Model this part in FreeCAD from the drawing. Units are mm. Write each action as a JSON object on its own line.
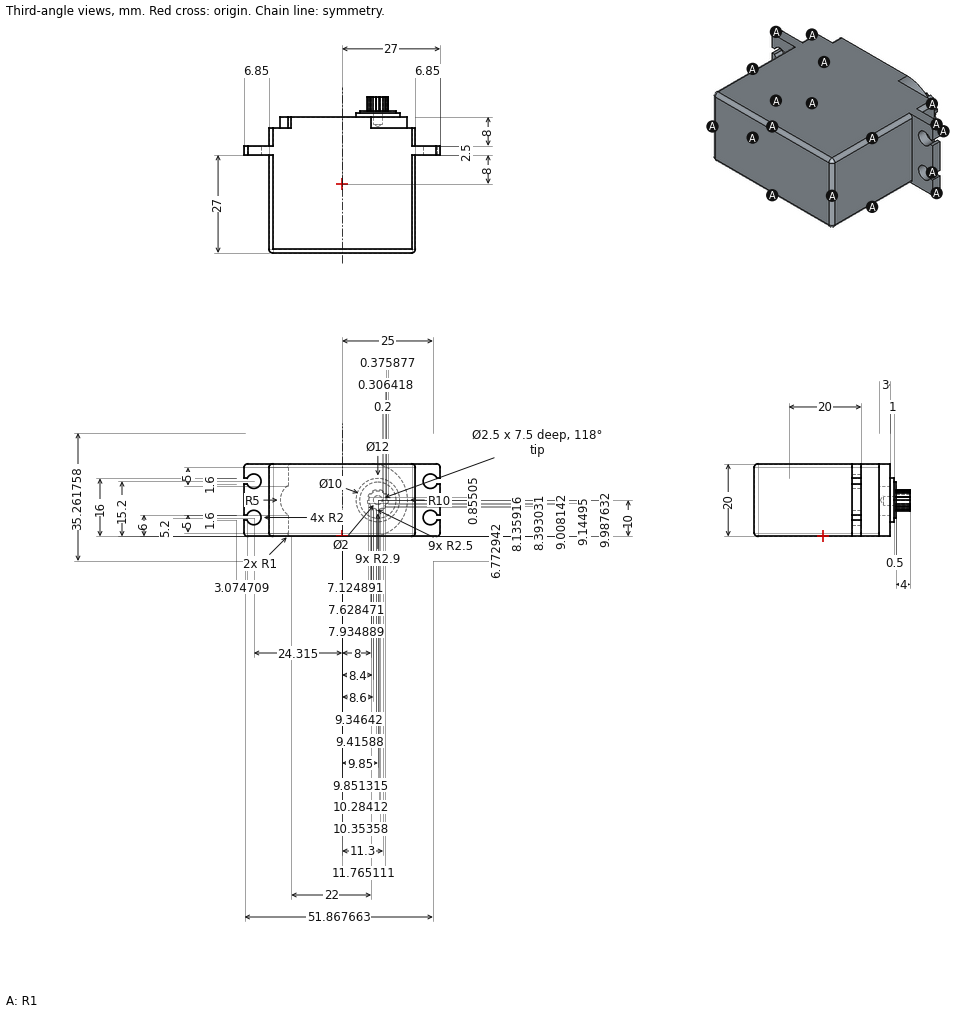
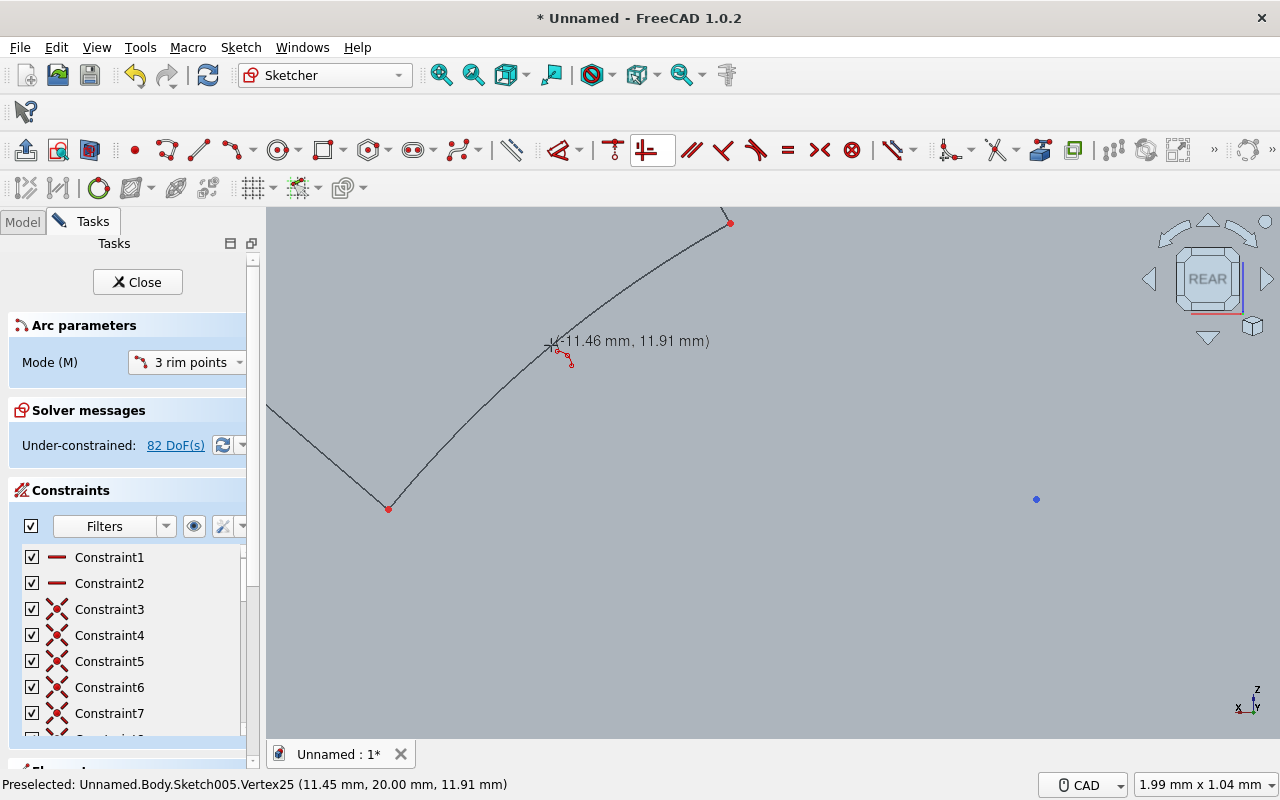
{"action": "scroll", "coordinate": [577, 333], "scroll_direction": "down", "scroll_amount": 15}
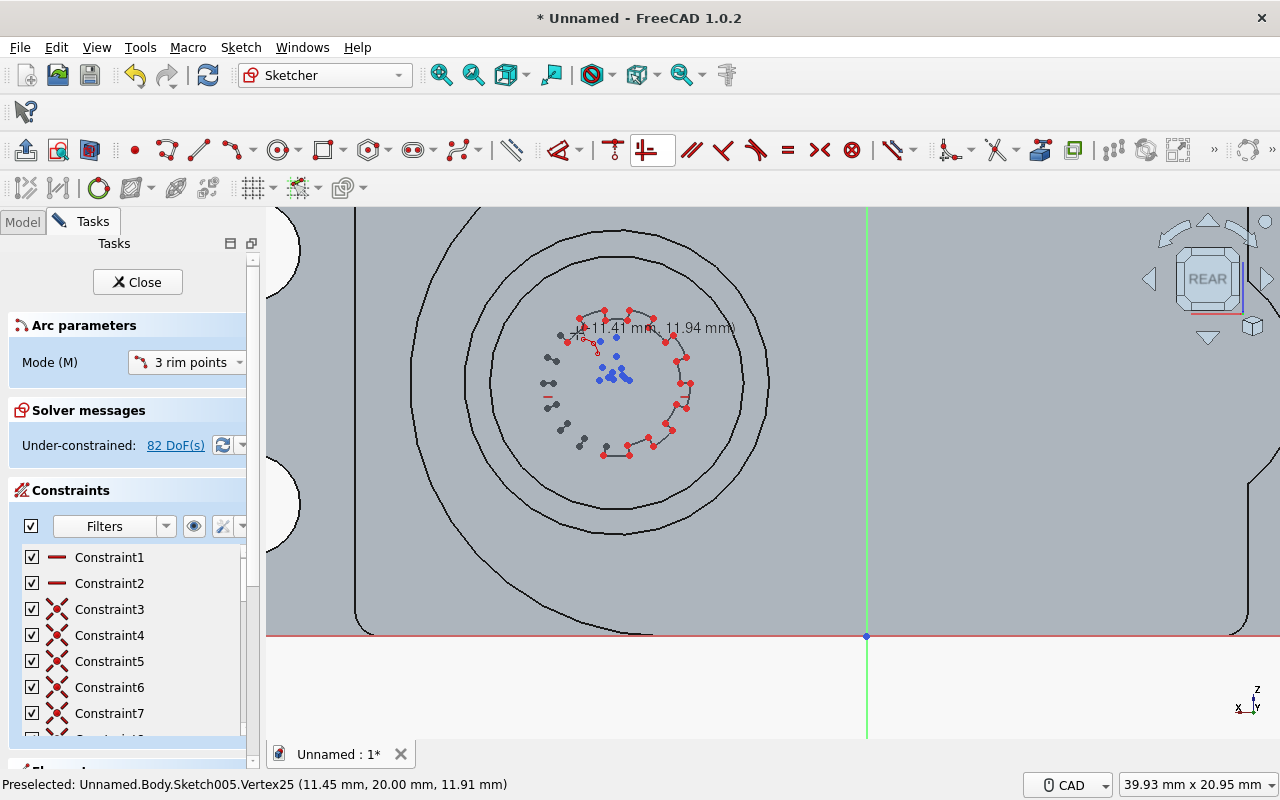
{"action": "scroll", "coordinate": [560, 335], "scroll_direction": "up", "scroll_amount": 6}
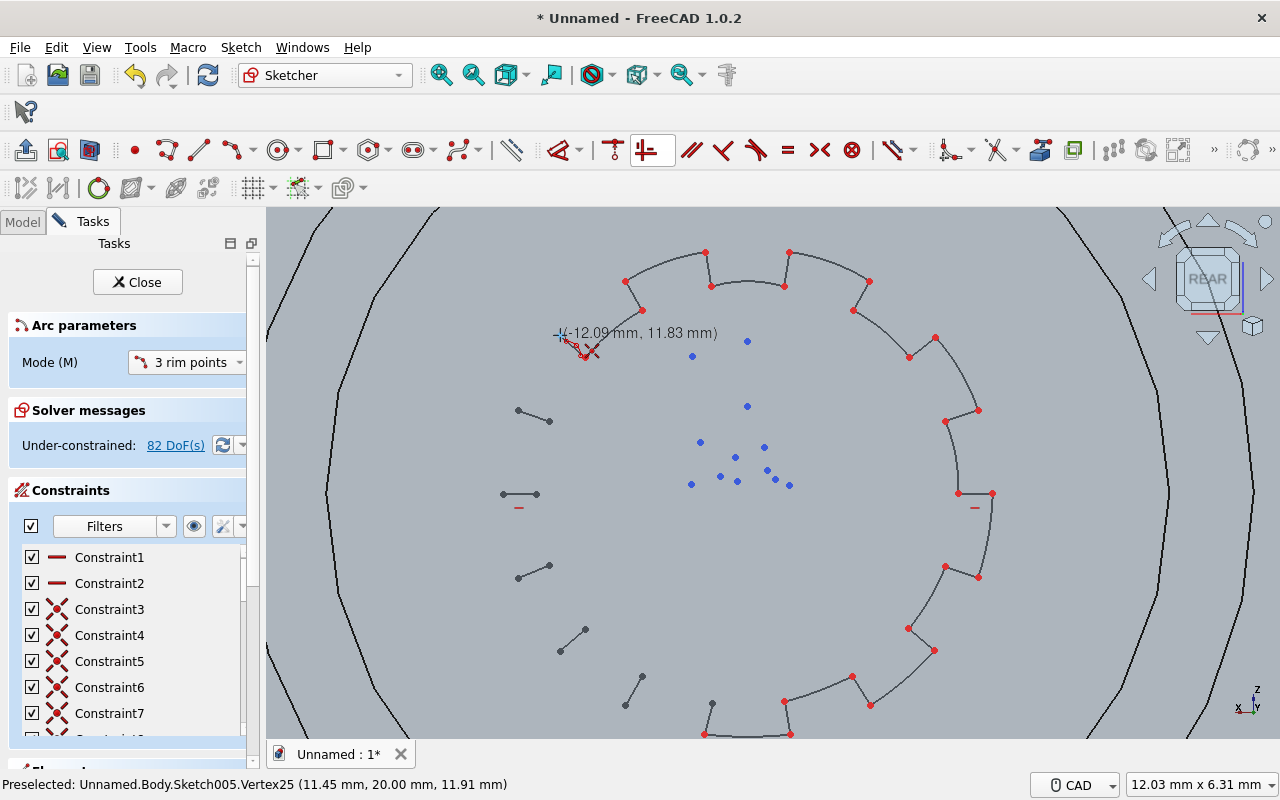
{"action": "left_click", "coordinate": [560, 336]}
{"action": "left_click", "coordinate": [518, 411]}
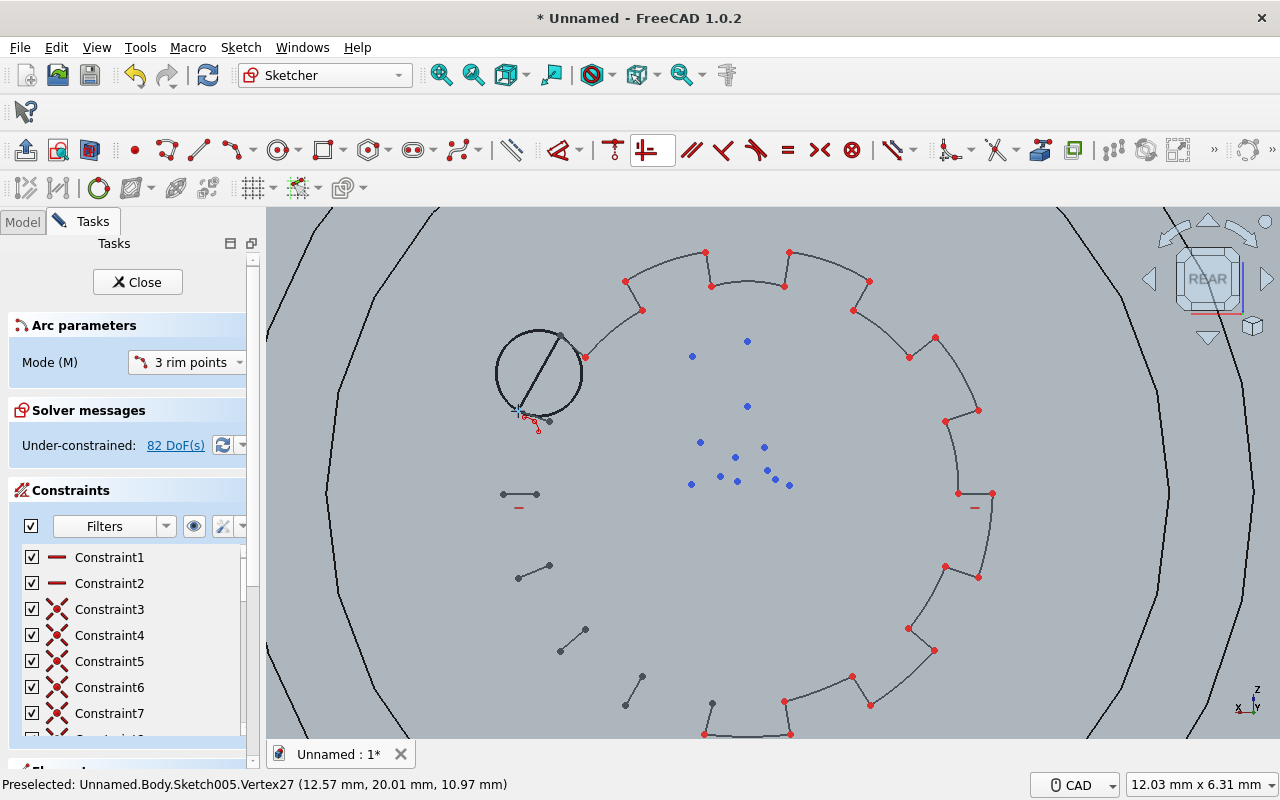
{"action": "scroll", "coordinate": [536, 370], "scroll_direction": "up", "scroll_amount": 8}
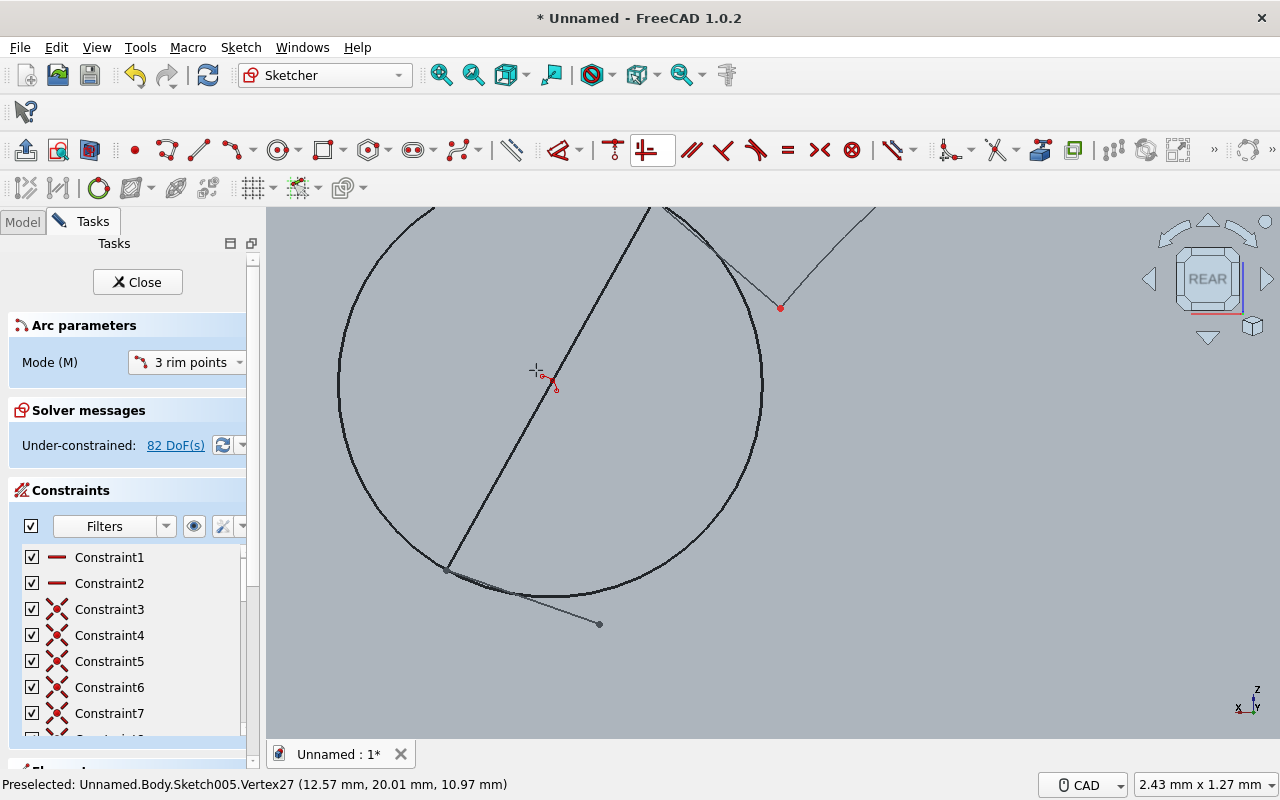
{"action": "left_click", "coordinate": [536, 368]}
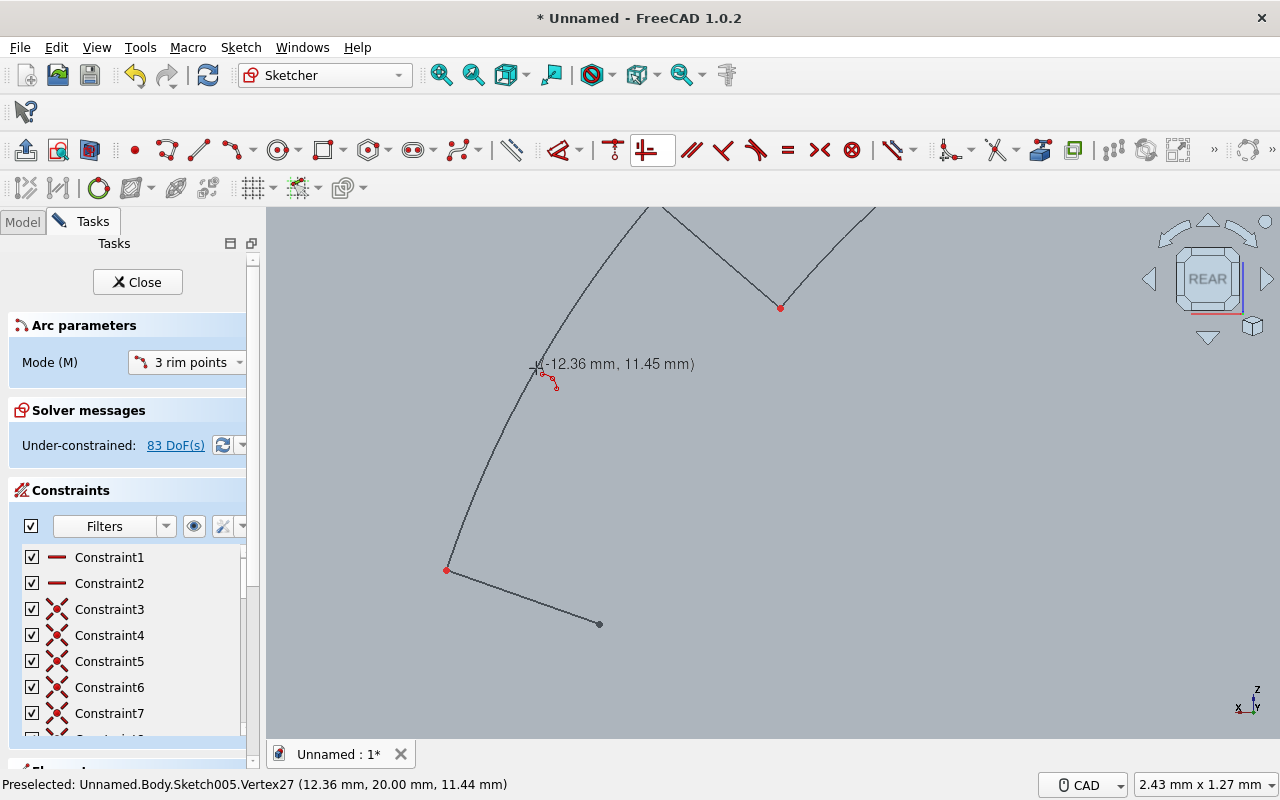
{"action": "scroll", "coordinate": [554, 344], "scroll_direction": "down", "scroll_amount": 14}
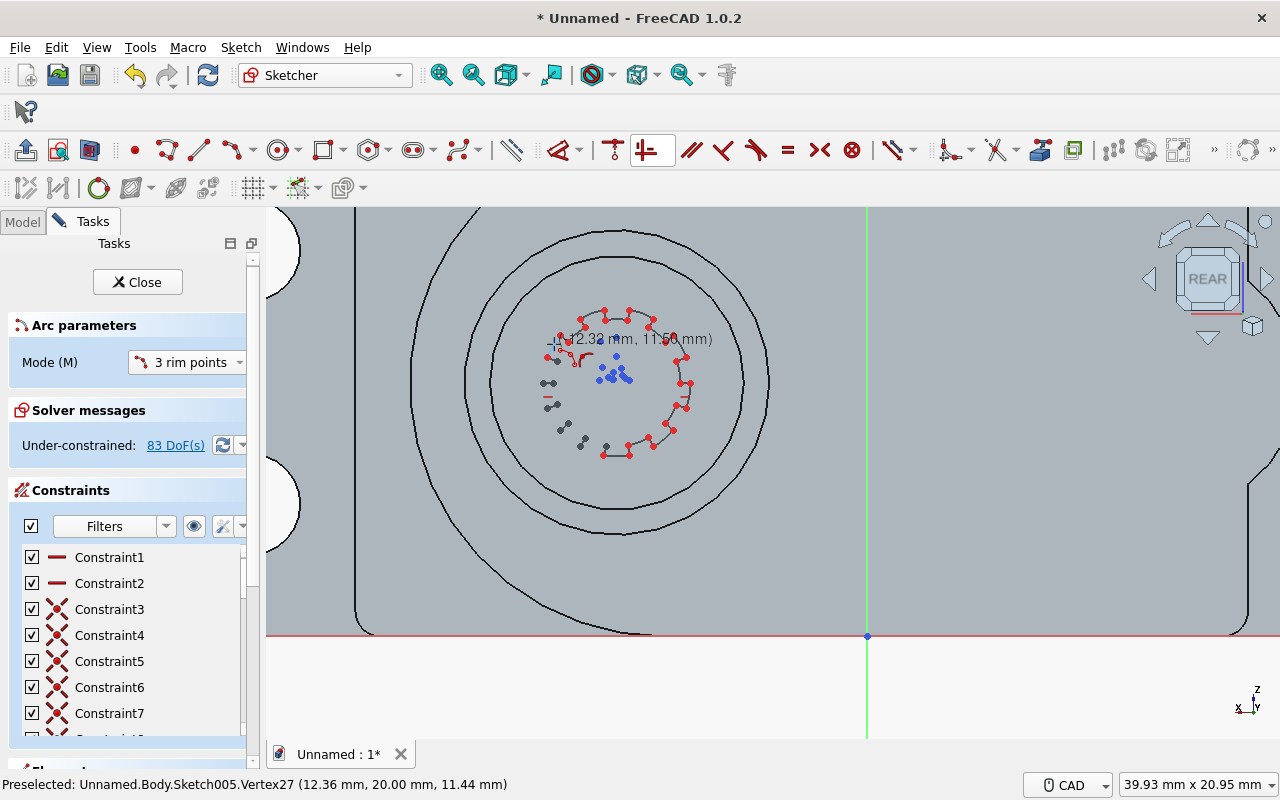
{"action": "scroll", "coordinate": [557, 361], "scroll_direction": "up", "scroll_amount": 6}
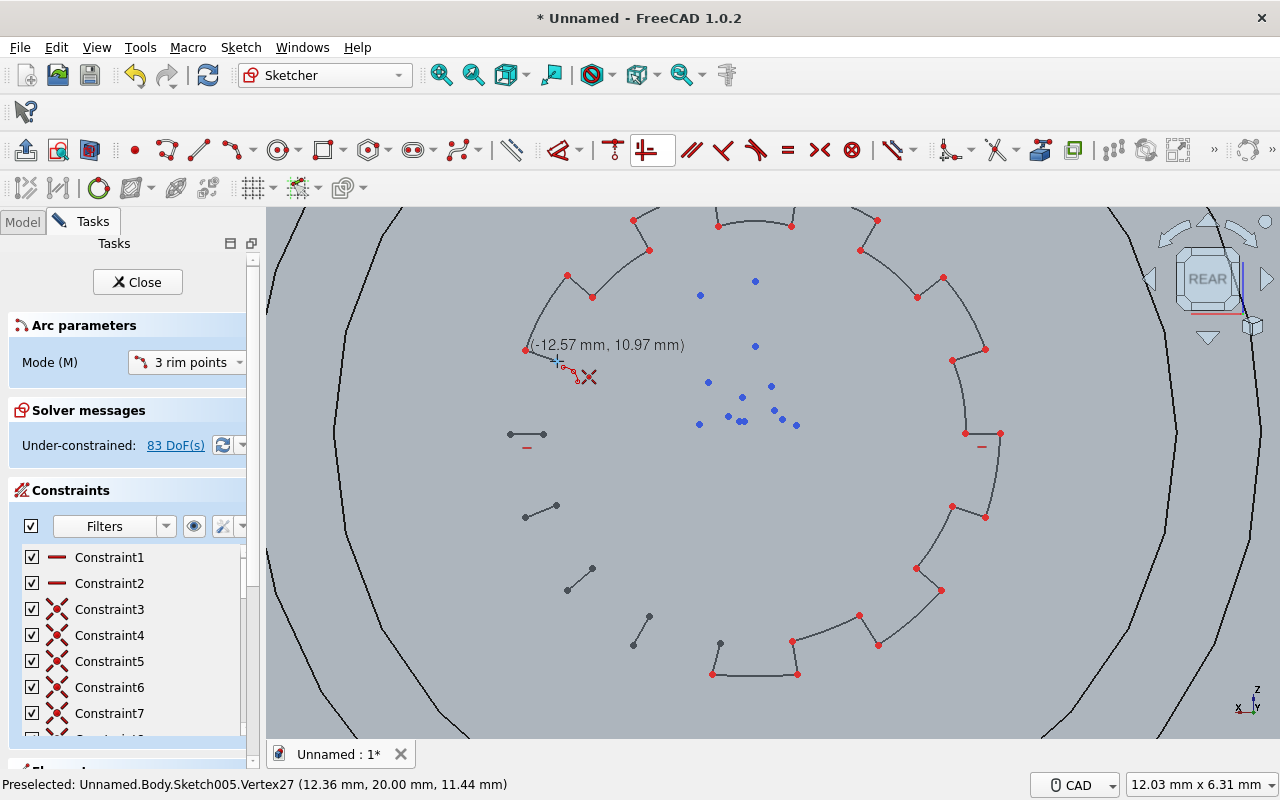
{"action": "left_click", "coordinate": [557, 361]}
{"action": "left_click", "coordinate": [544, 434]}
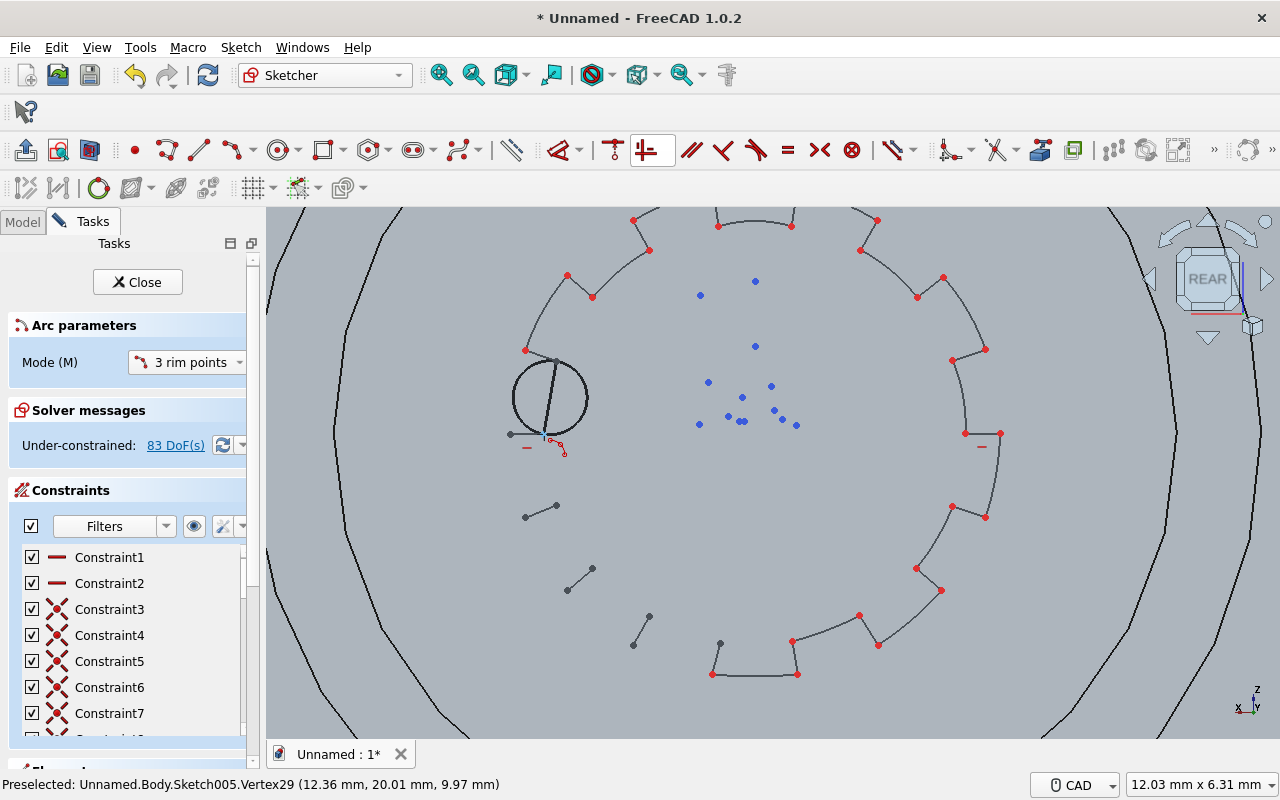
{"action": "scroll", "coordinate": [548, 395], "scroll_direction": "up", "scroll_amount": 9}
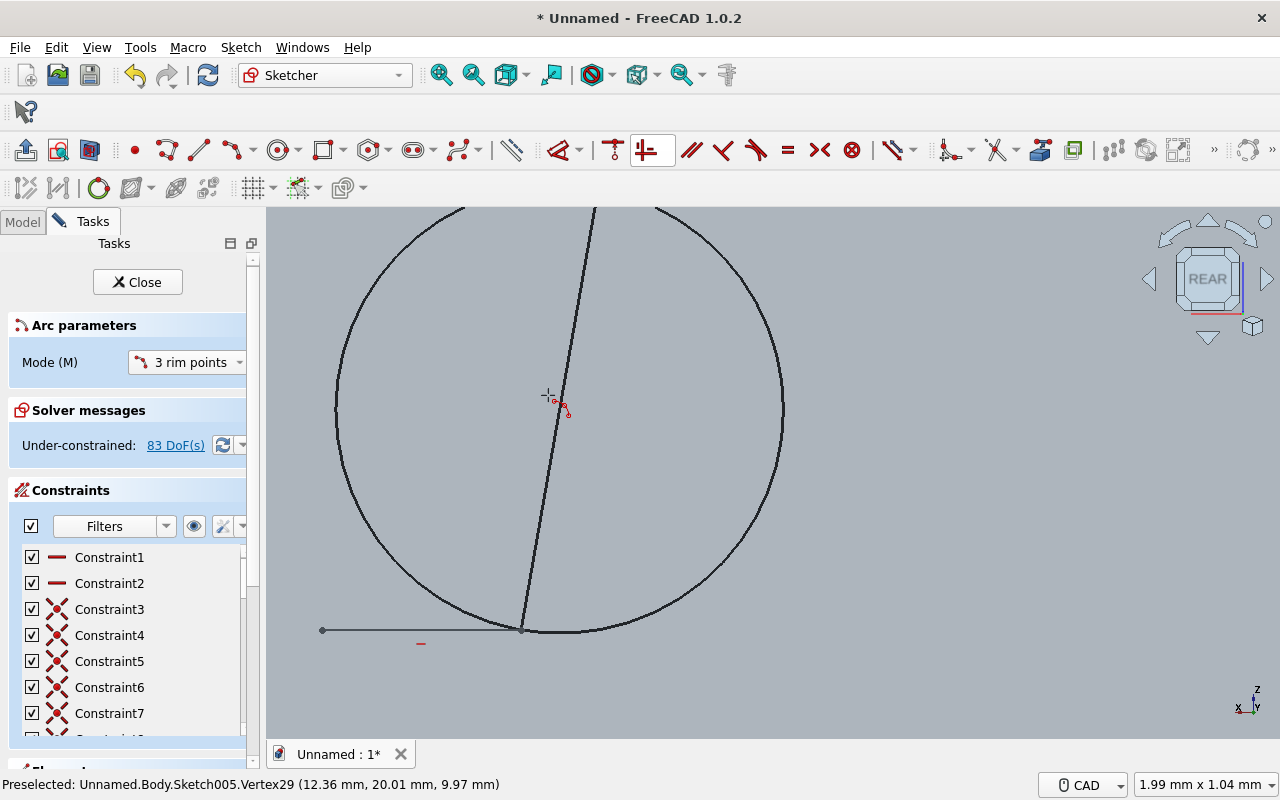
{"action": "left_click", "coordinate": [545, 394]}